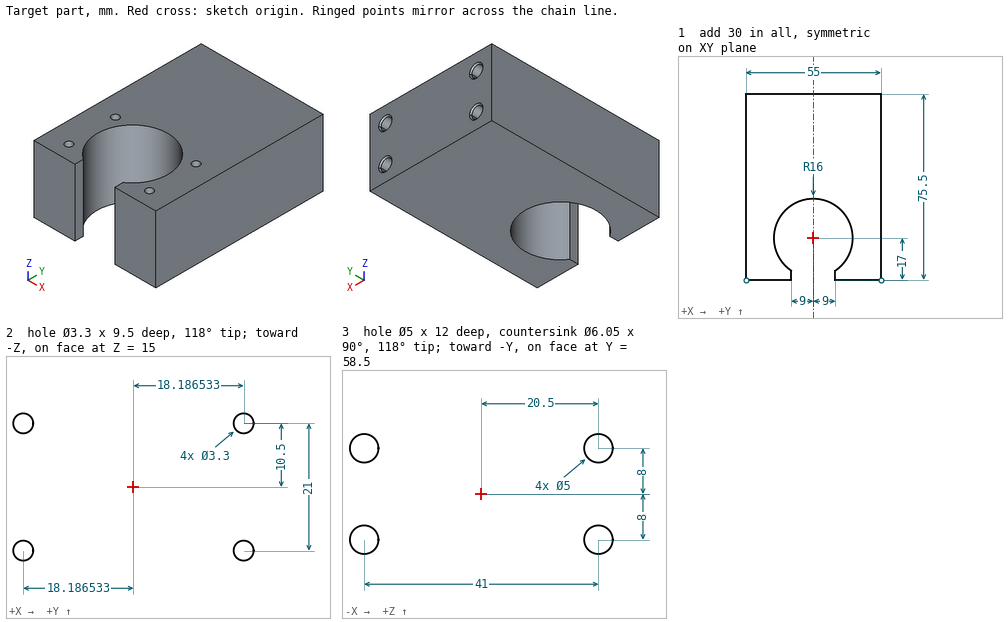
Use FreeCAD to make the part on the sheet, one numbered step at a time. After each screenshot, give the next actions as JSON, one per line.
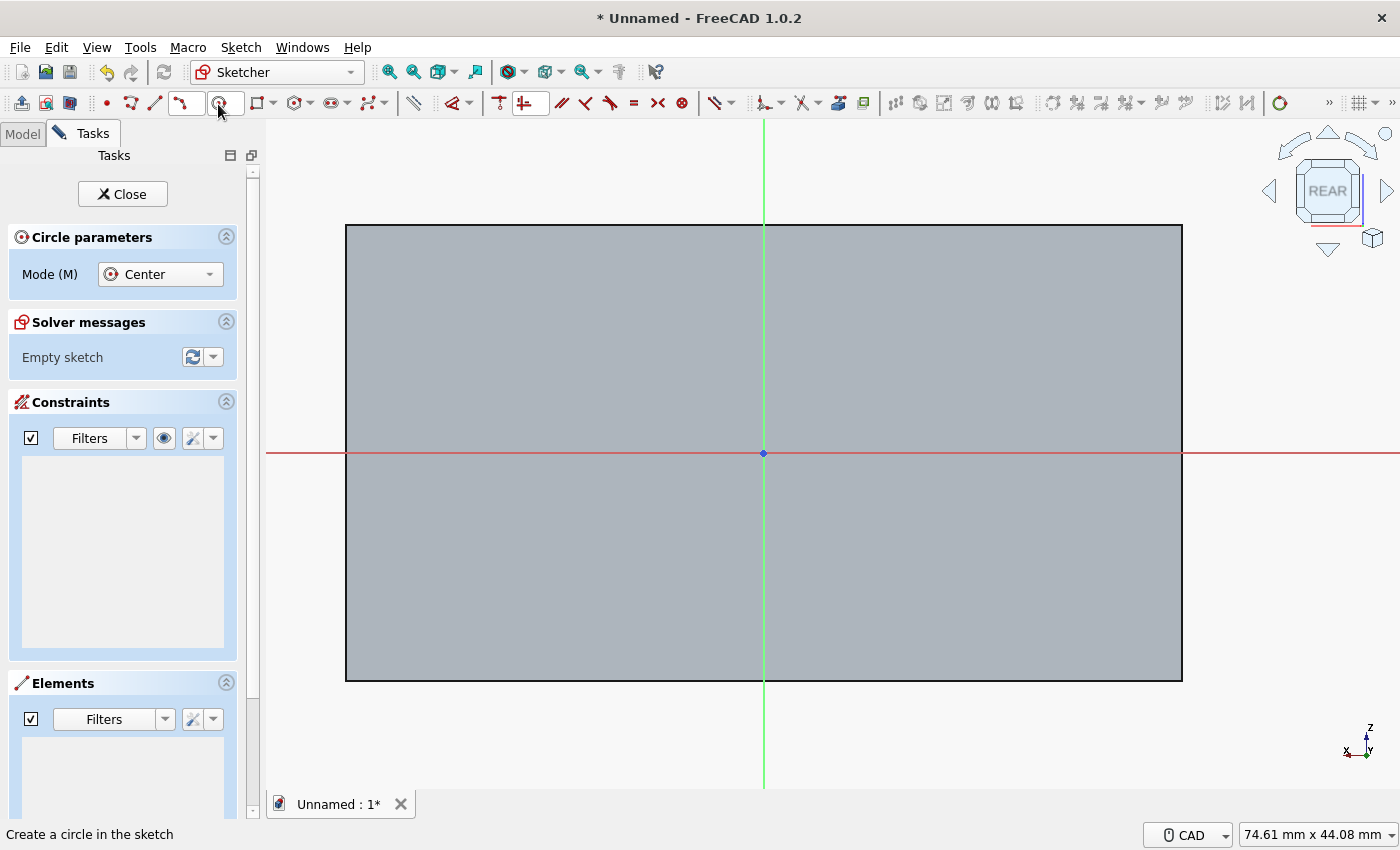
{"action": "left_click", "coordinate": [1075, 332]}
{"action": "left_click", "coordinate": [1102, 305]}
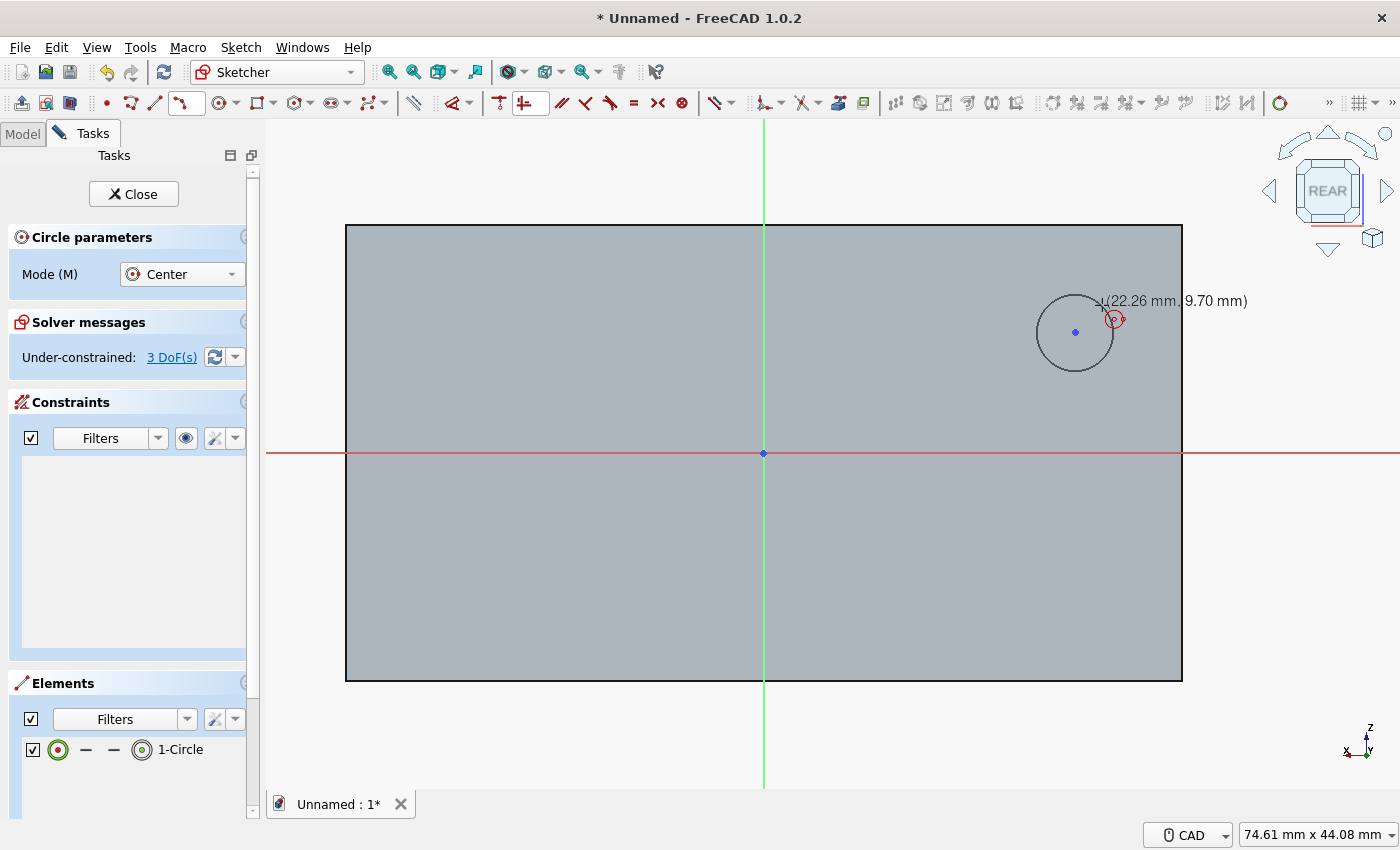
{"action": "left_click", "coordinate": [1075, 575]}
{"action": "left_click", "coordinate": [1102, 548]}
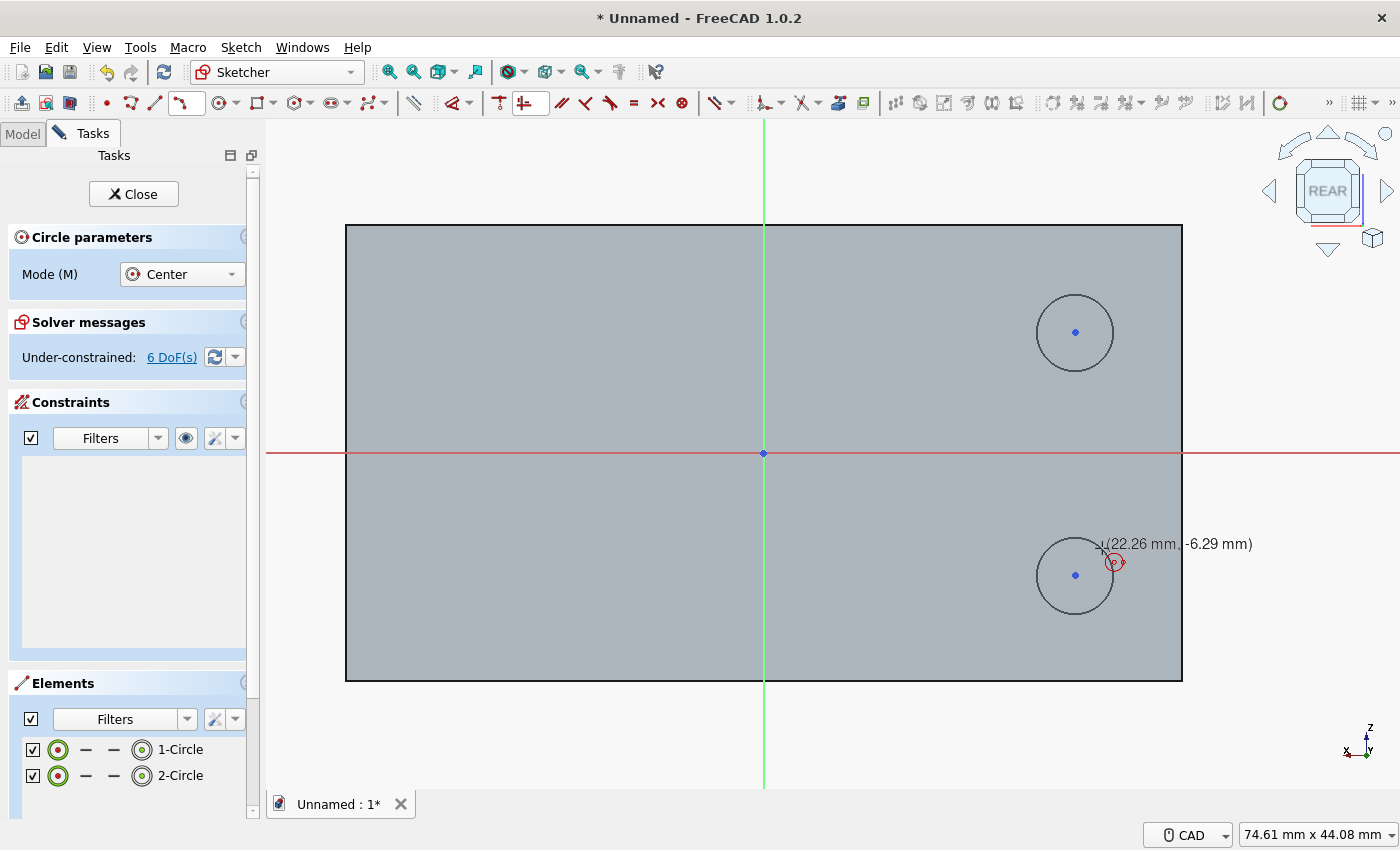
{"action": "left_click", "coordinate": [452, 575]}
{"action": "left_click", "coordinate": [479, 548]}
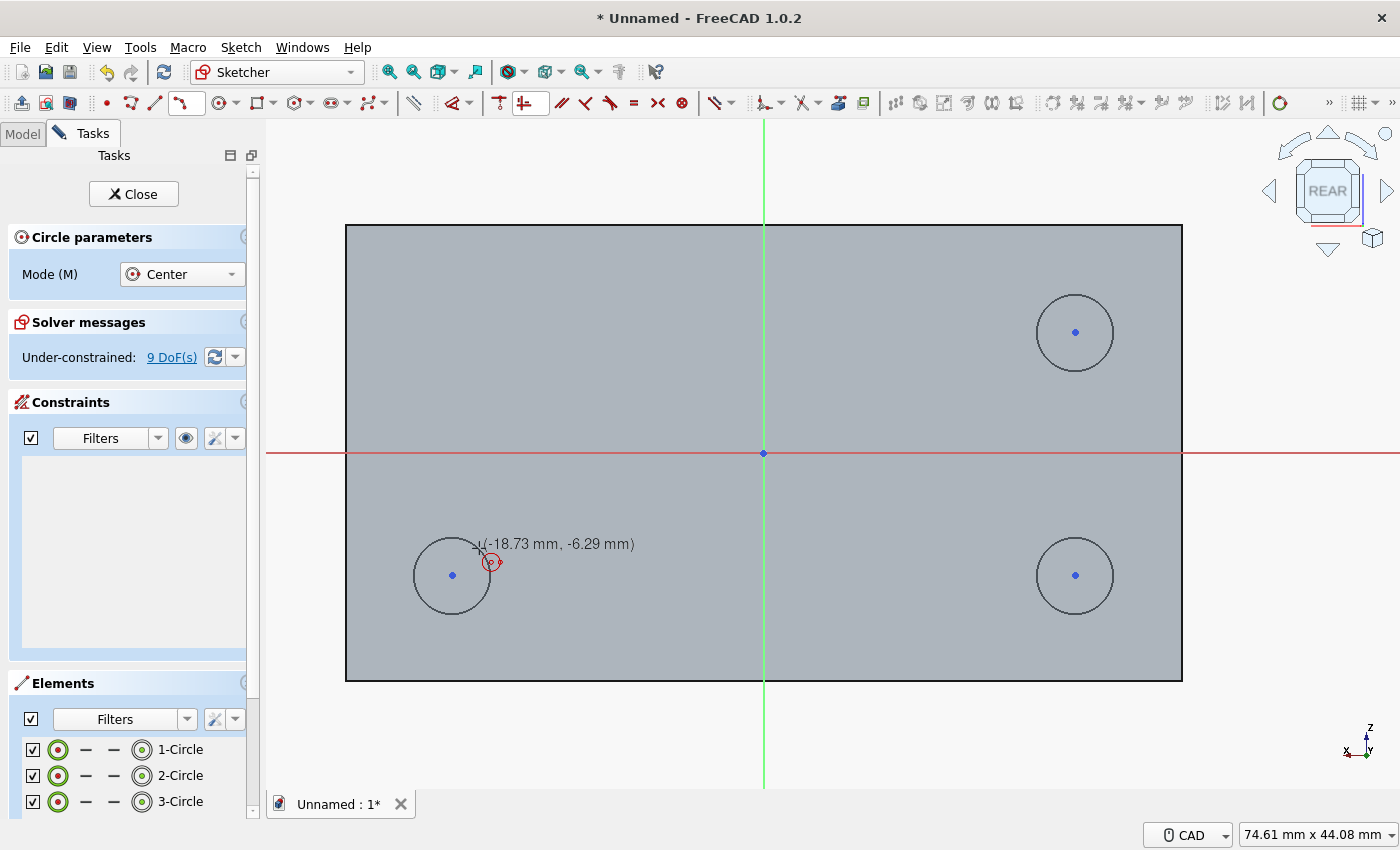
{"action": "left_click", "coordinate": [452, 332]}
{"action": "left_click", "coordinate": [479, 305]}
{"action": "key", "text": "Escape"}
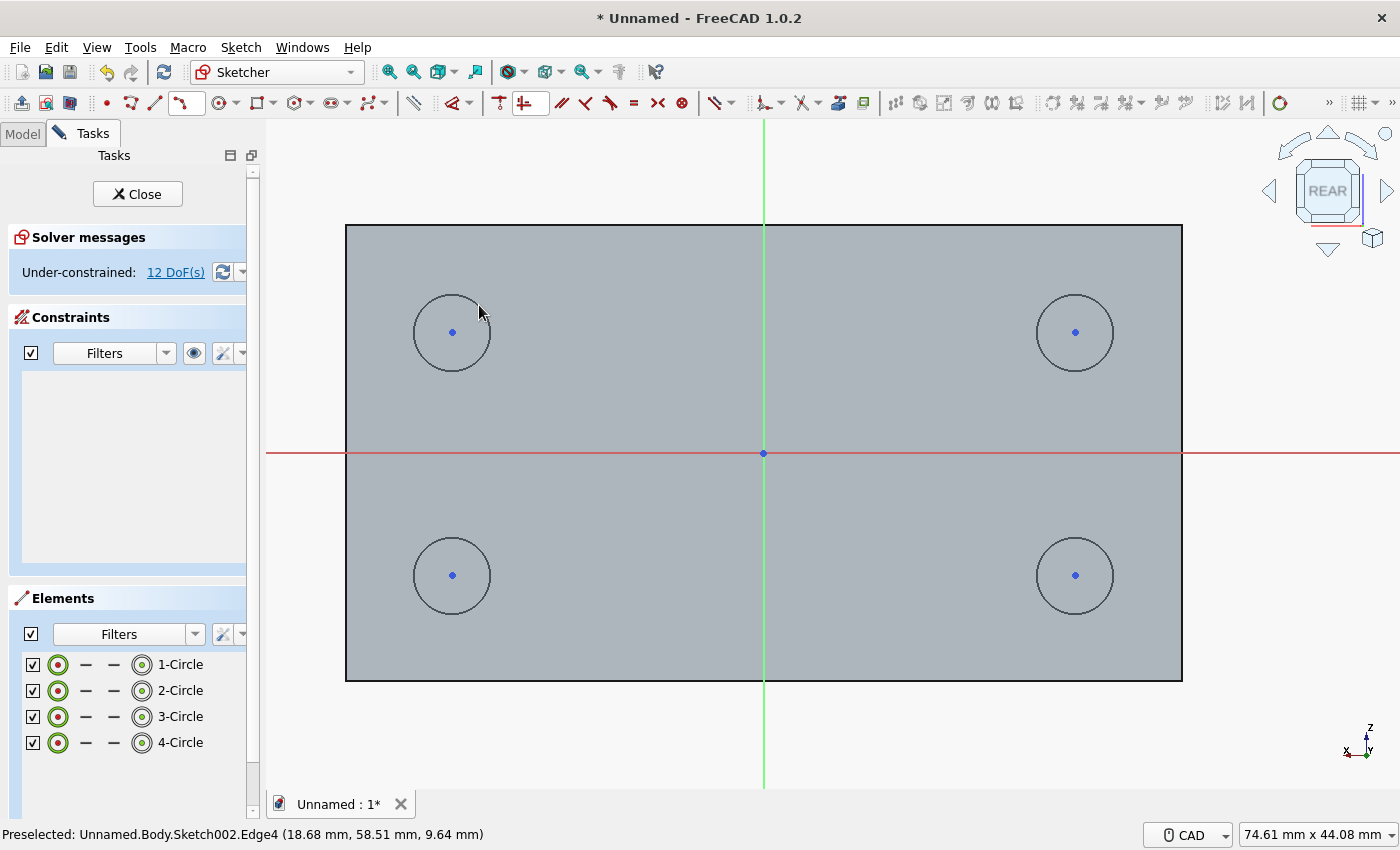
{"action": "left_click", "coordinate": [1102, 306]}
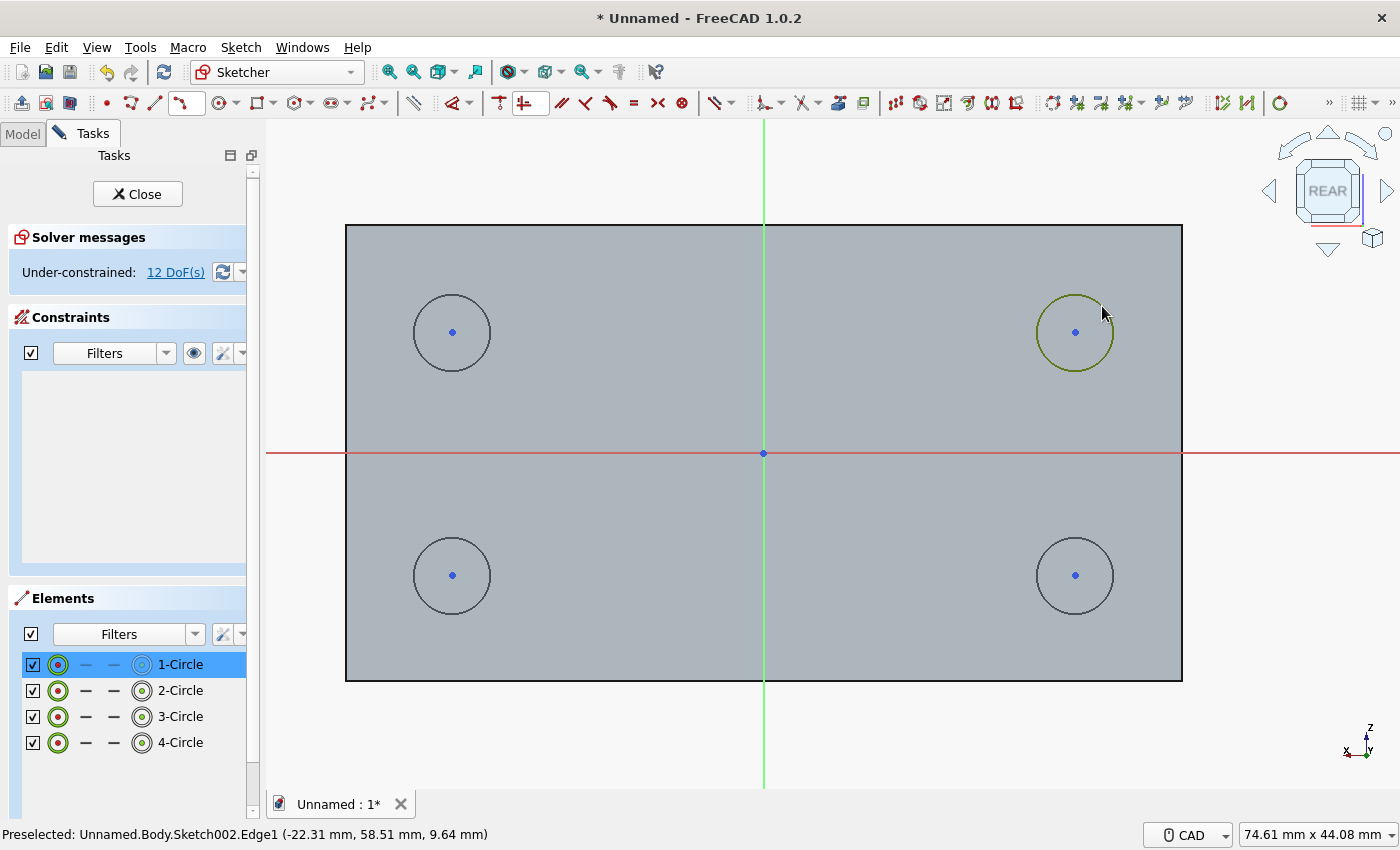
{"action": "left_click", "coordinate": [1102, 549]}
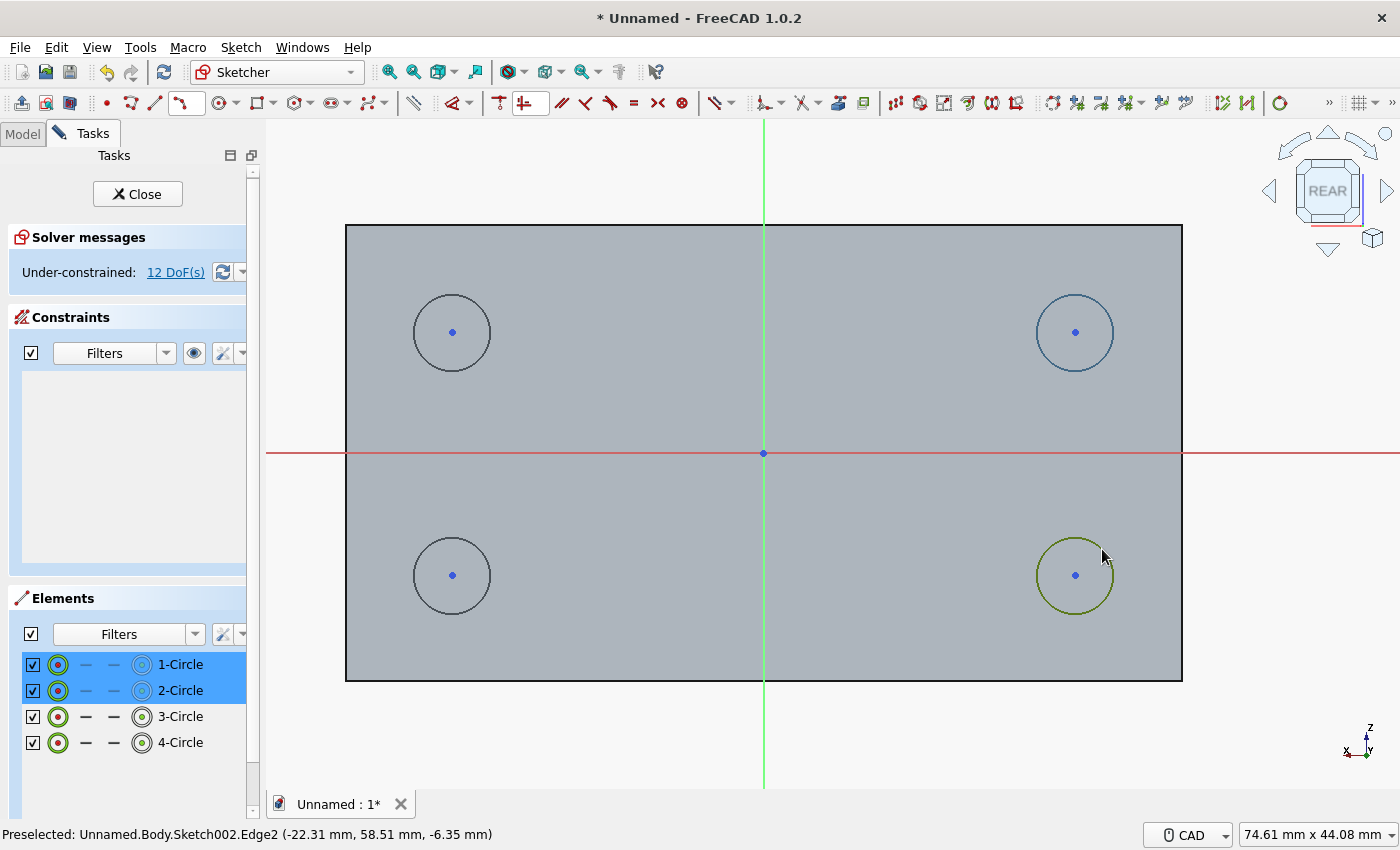
{"action": "left_click", "coordinate": [479, 549]}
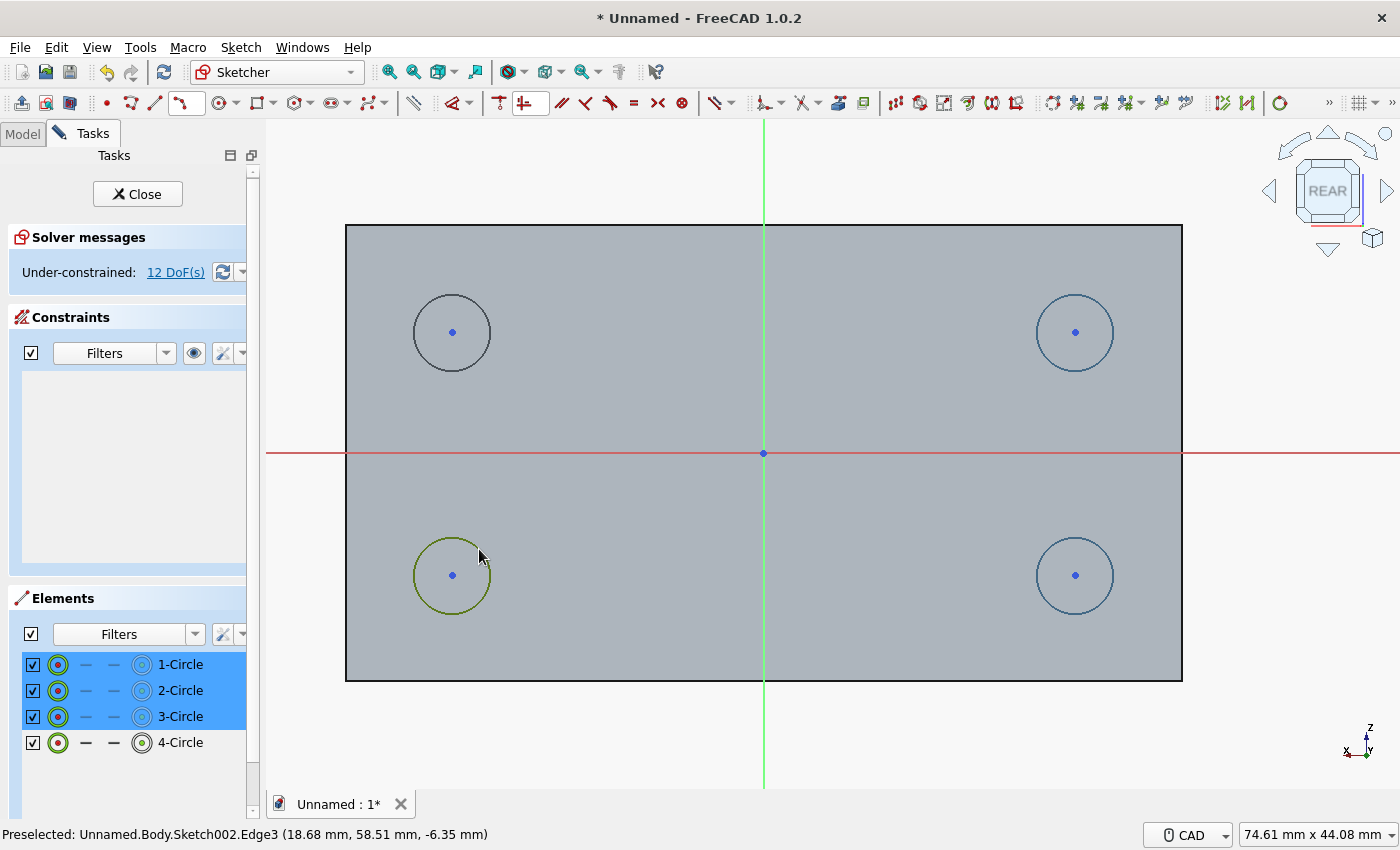
{"action": "left_click", "coordinate": [479, 306]}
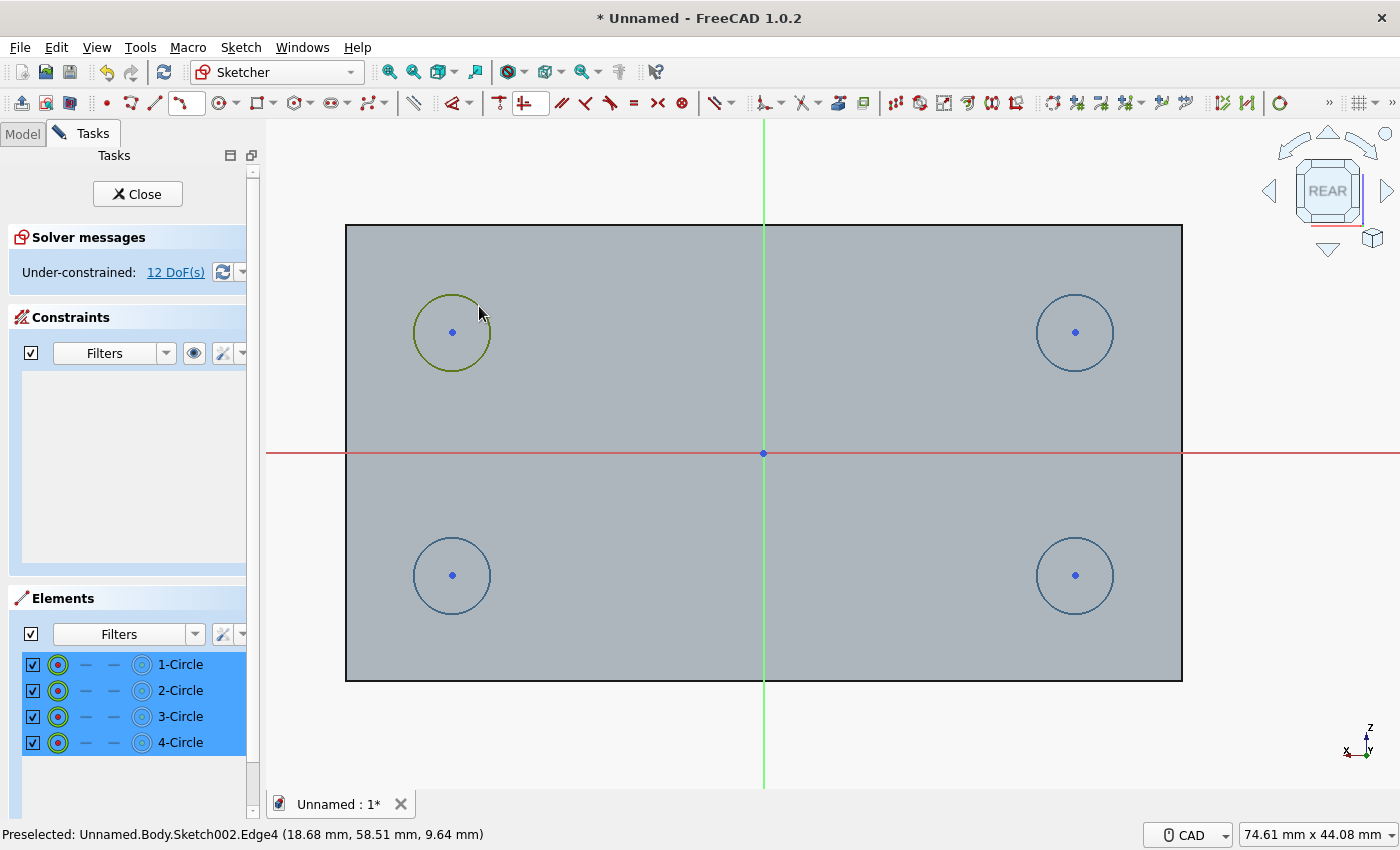
{"action": "left_click", "coordinate": [634, 104]}